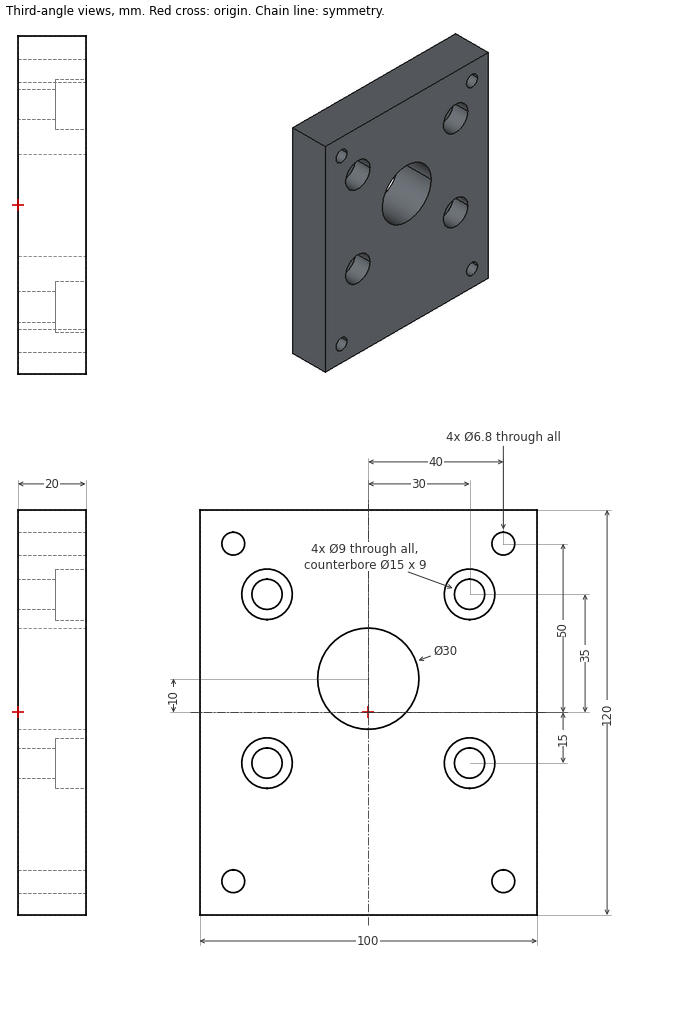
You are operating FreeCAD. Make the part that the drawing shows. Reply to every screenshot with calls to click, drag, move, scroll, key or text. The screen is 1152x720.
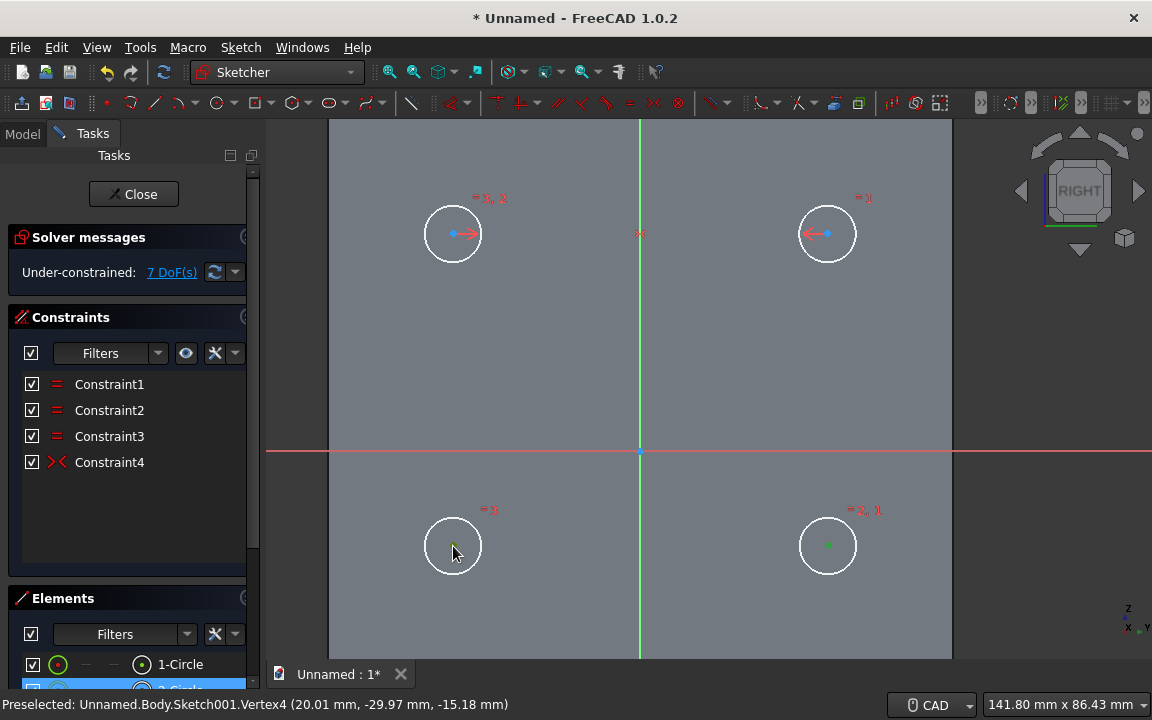
click(640, 596)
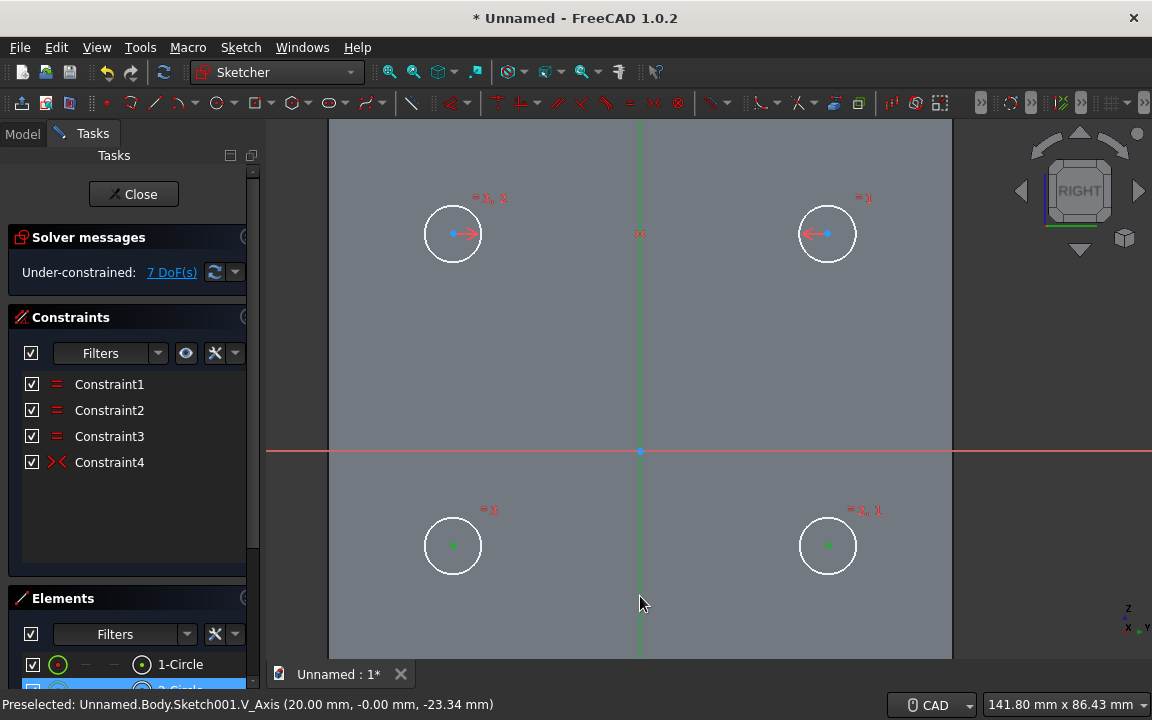
click(654, 104)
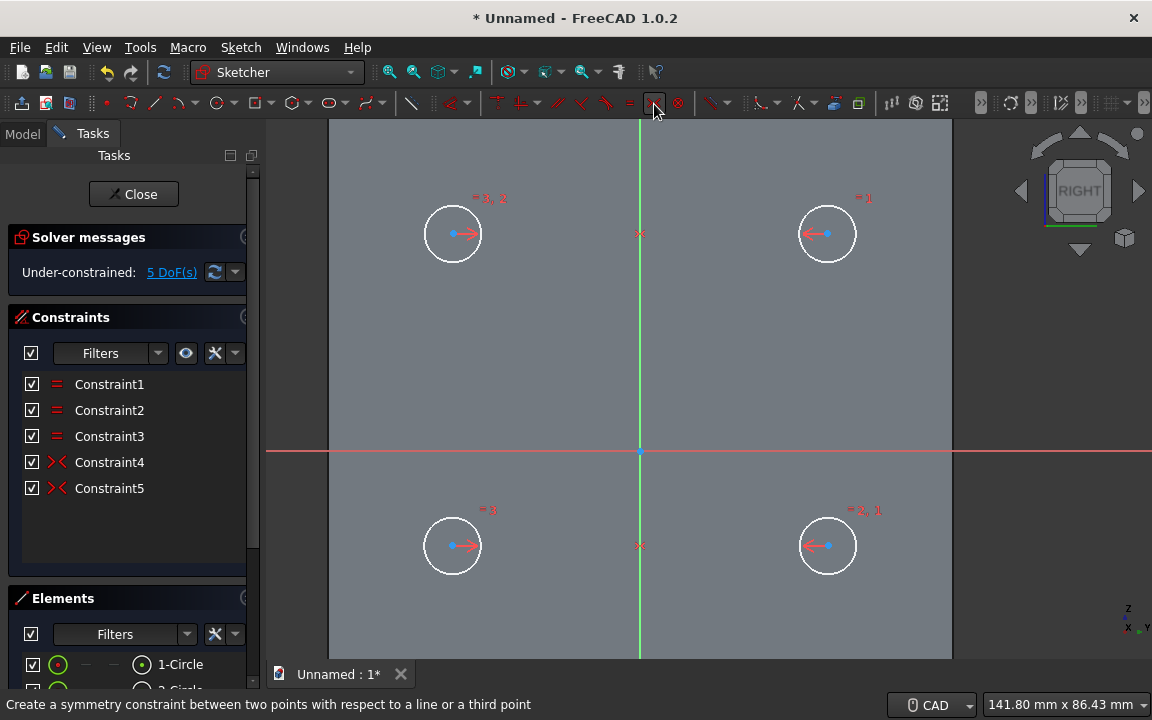
click(450, 104)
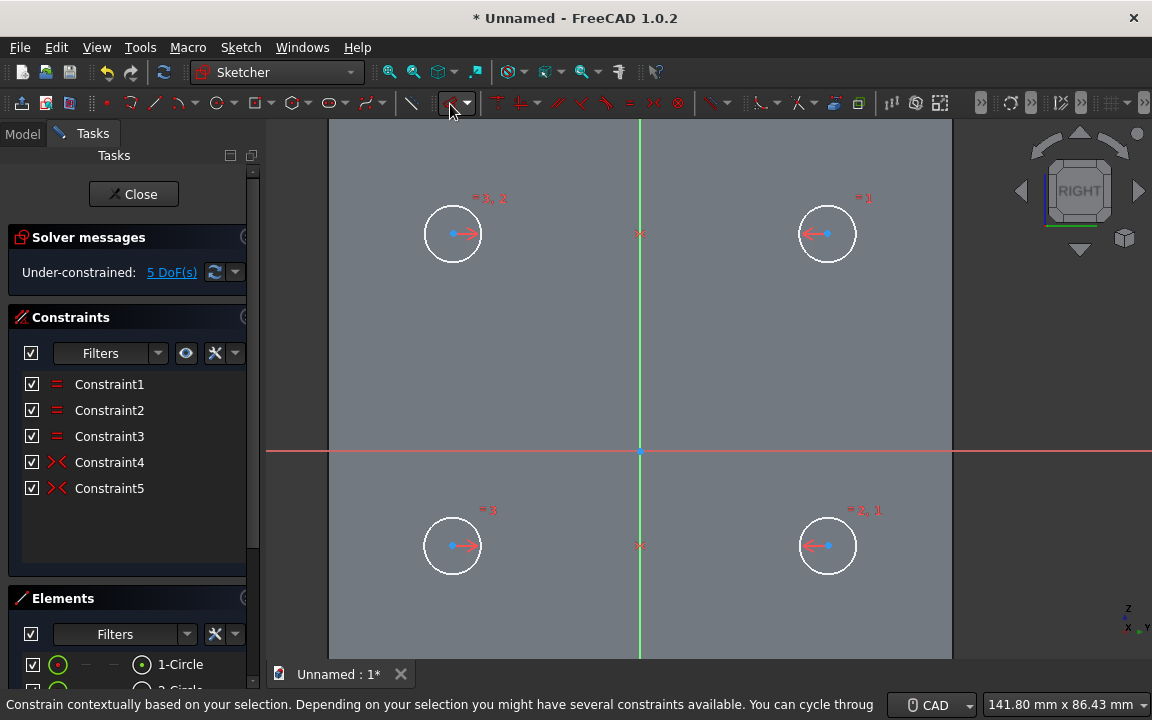
click(847, 214)
click(869, 191)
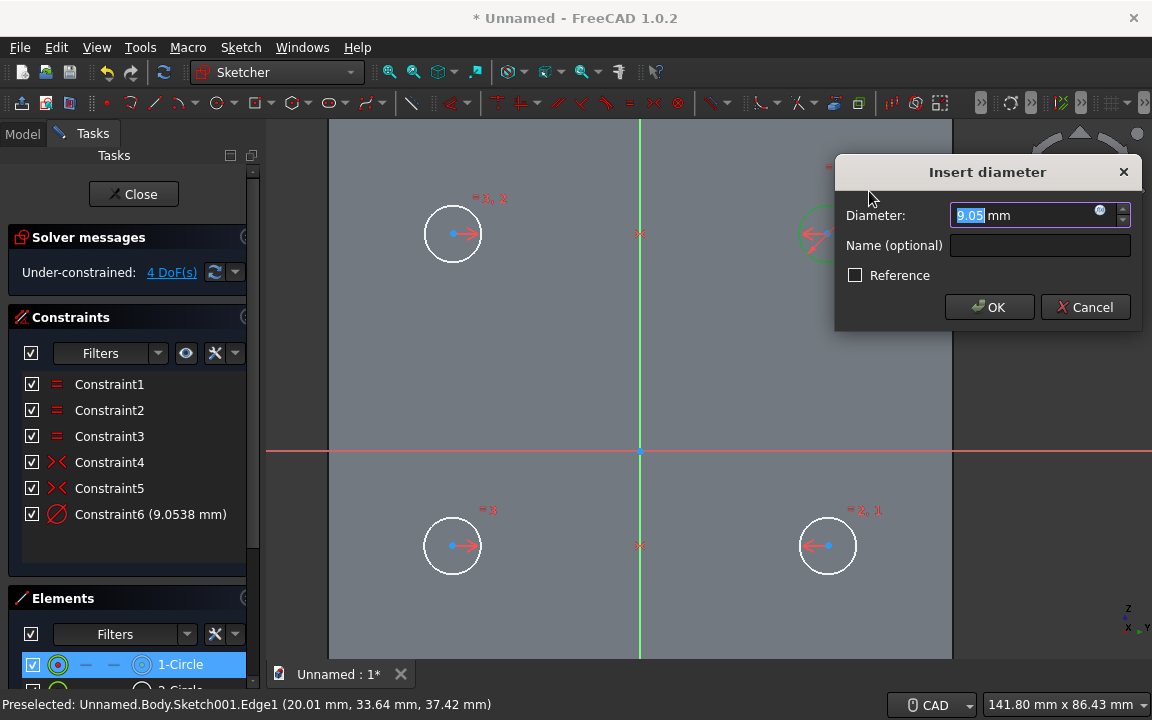
text(9)
key(Return)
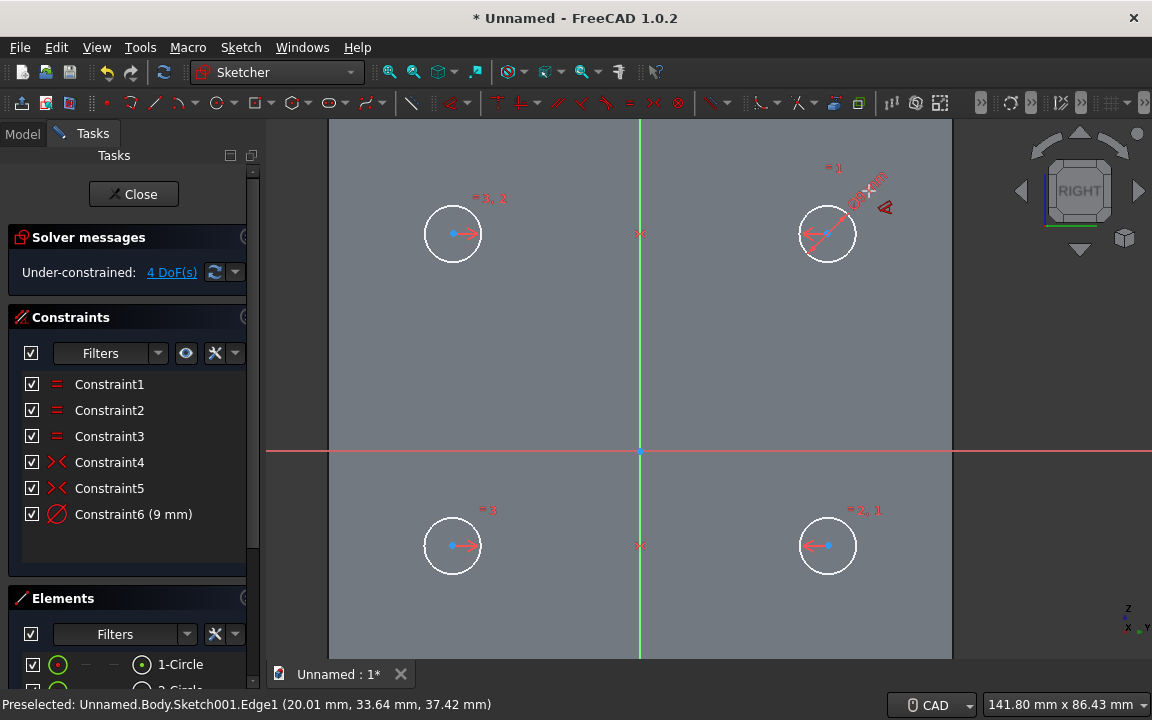
click(828, 234)
click(734, 200)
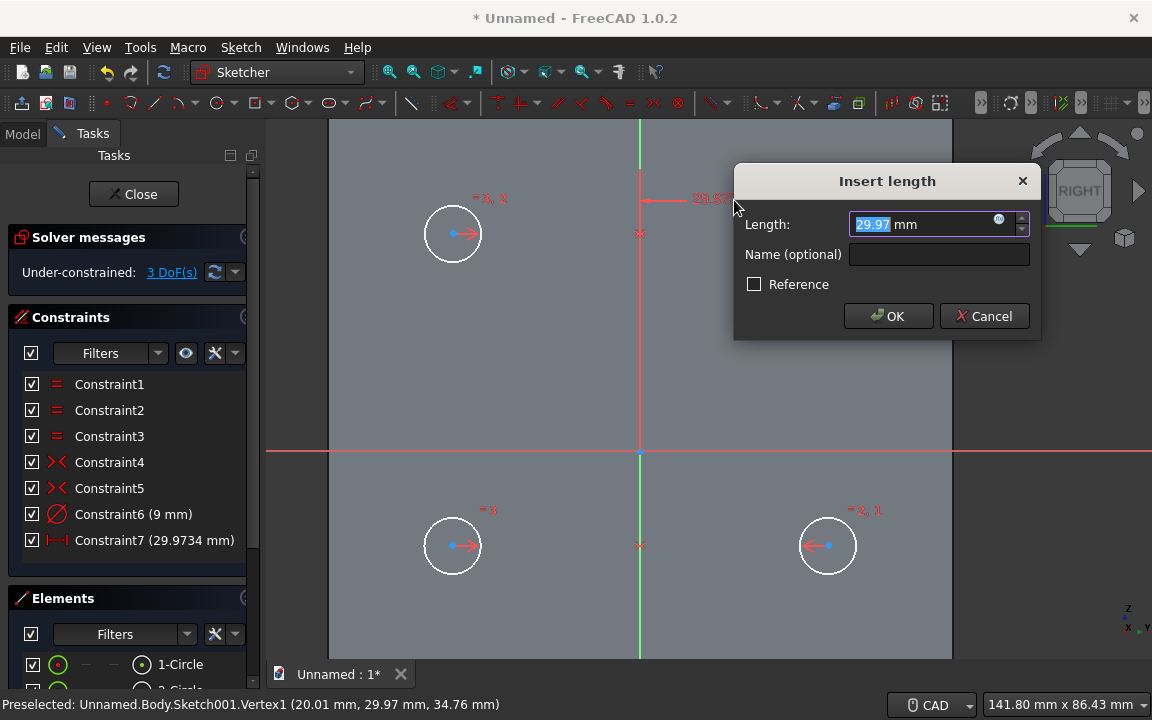
text(30)
key(Return)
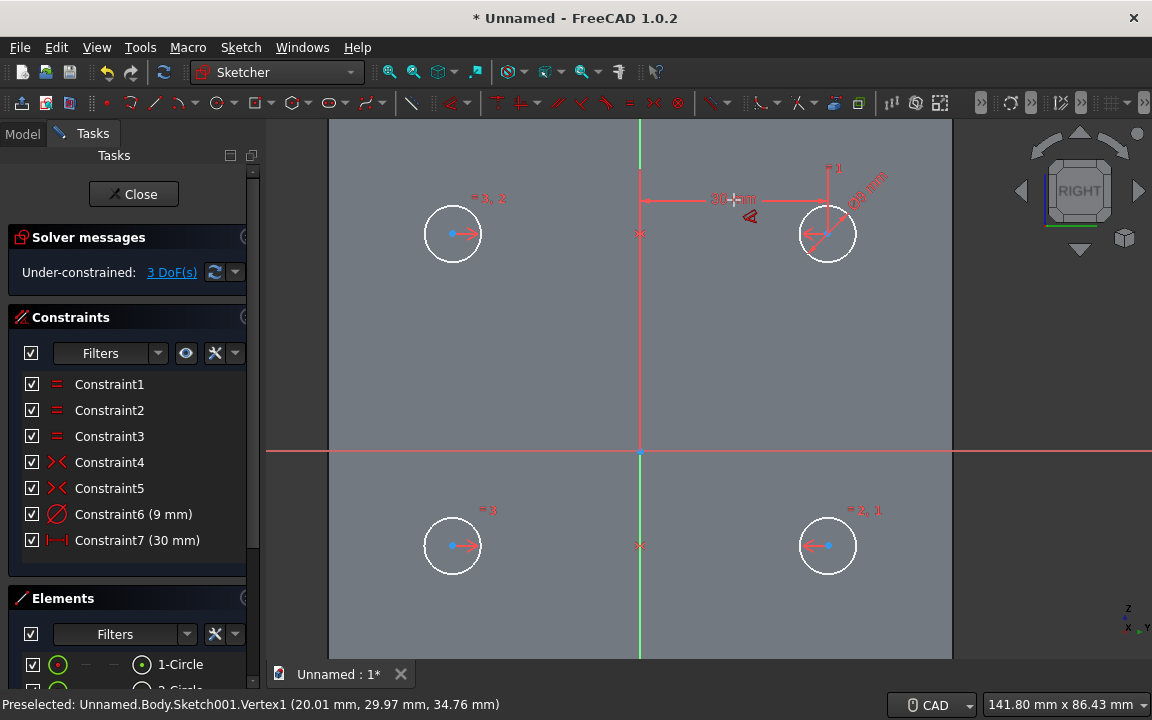
click(828, 234)
click(862, 343)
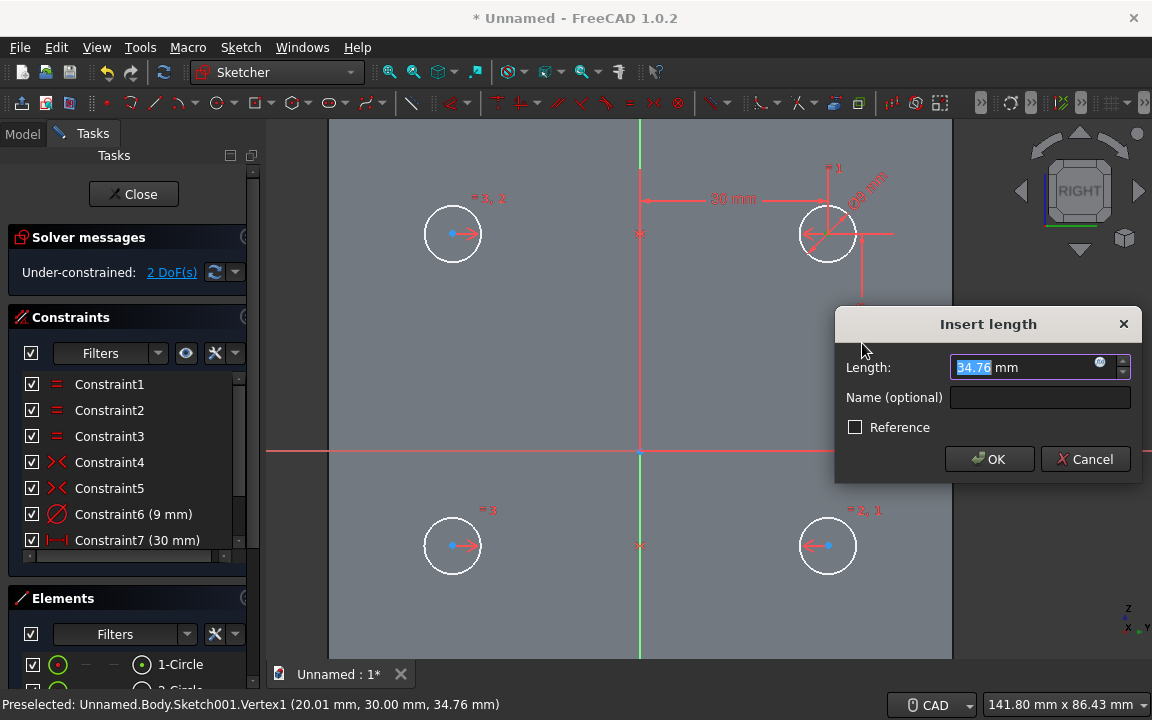
text(35)
key(Return)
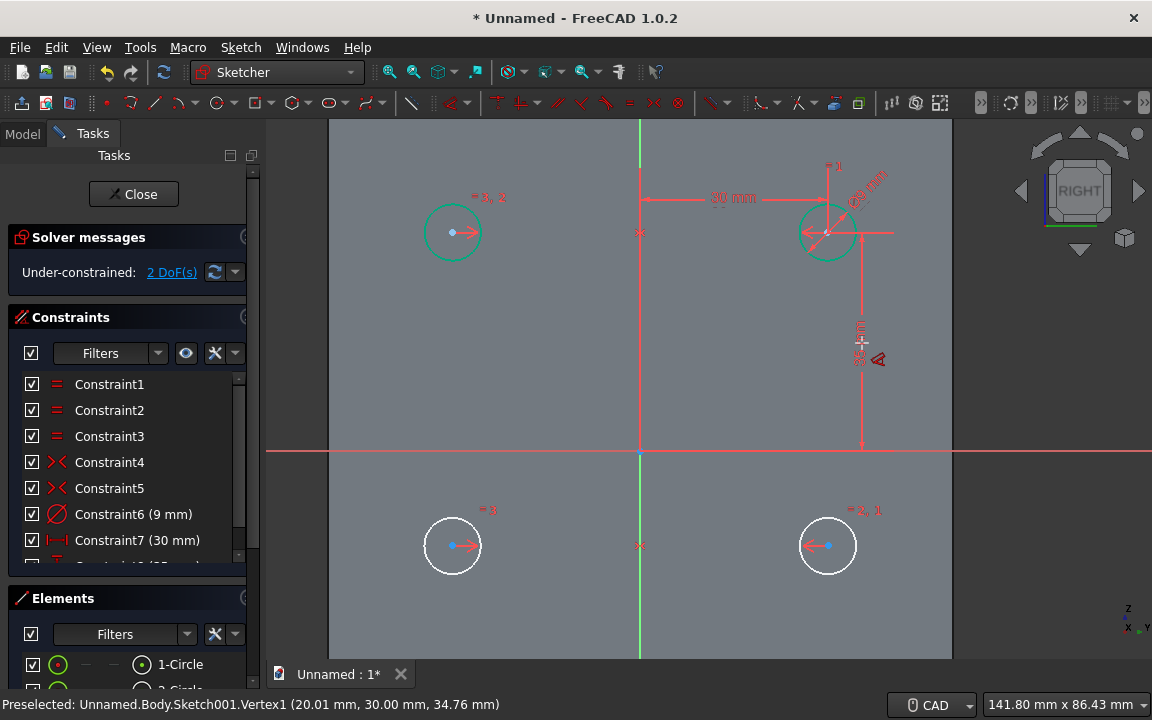
click(828, 546)
click(734, 580)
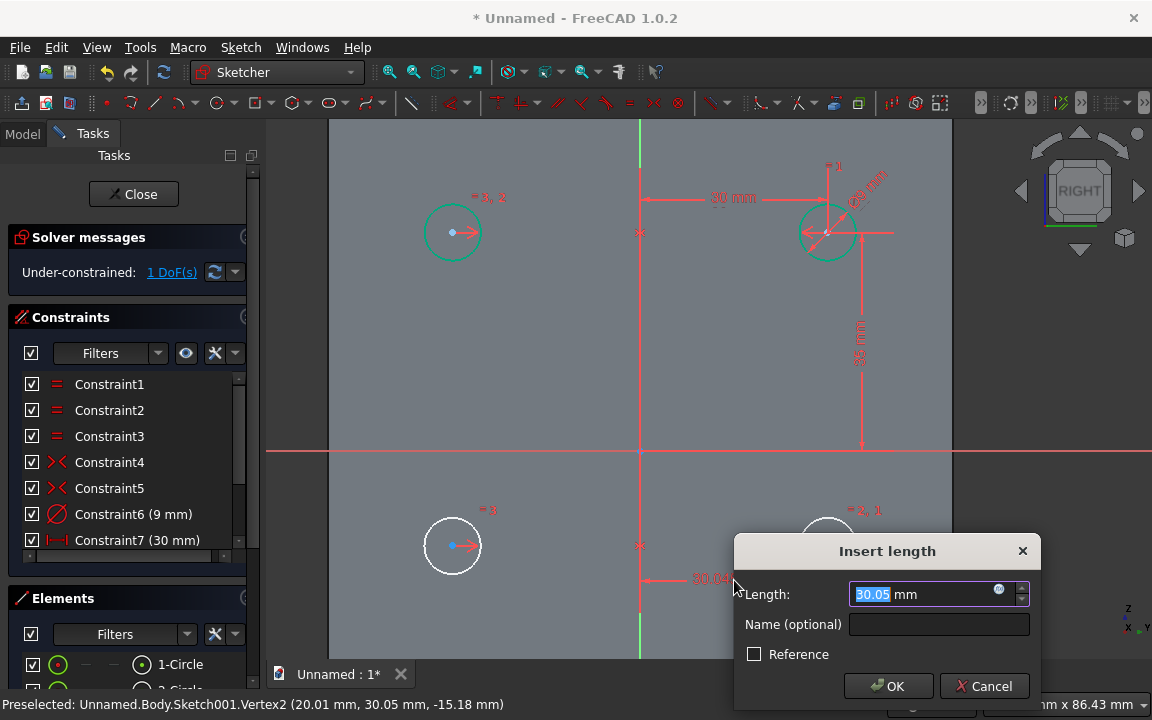
text(30)
key(Return)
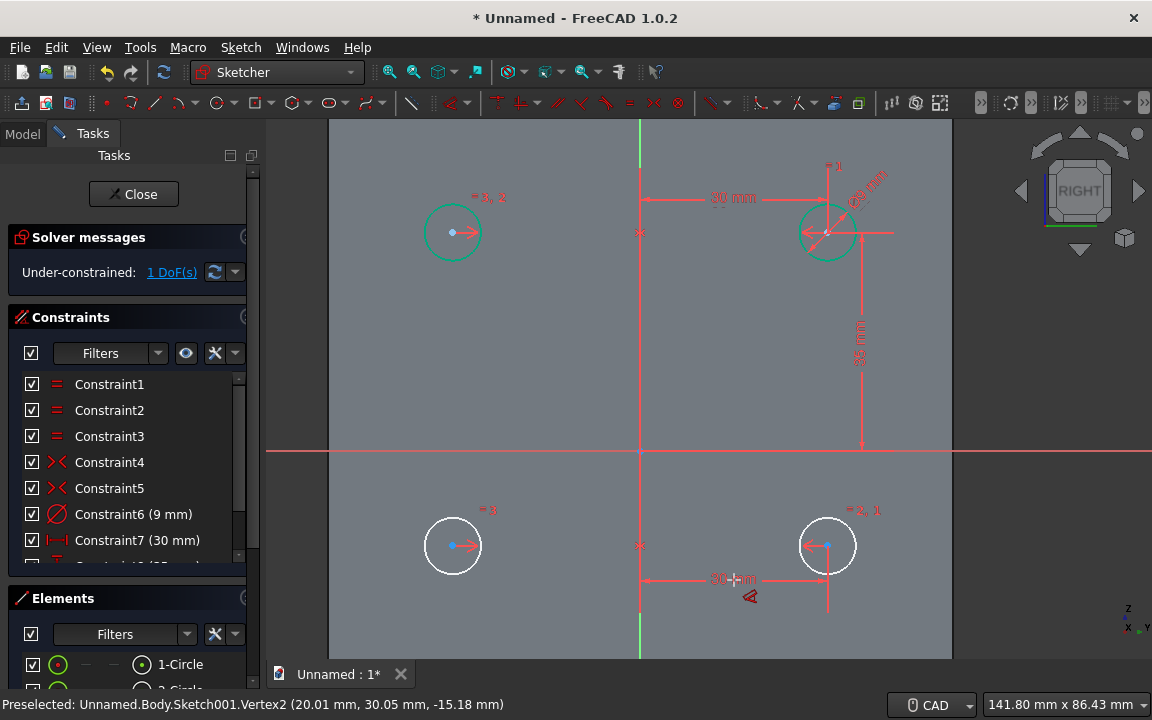
click(828, 546)
click(862, 499)